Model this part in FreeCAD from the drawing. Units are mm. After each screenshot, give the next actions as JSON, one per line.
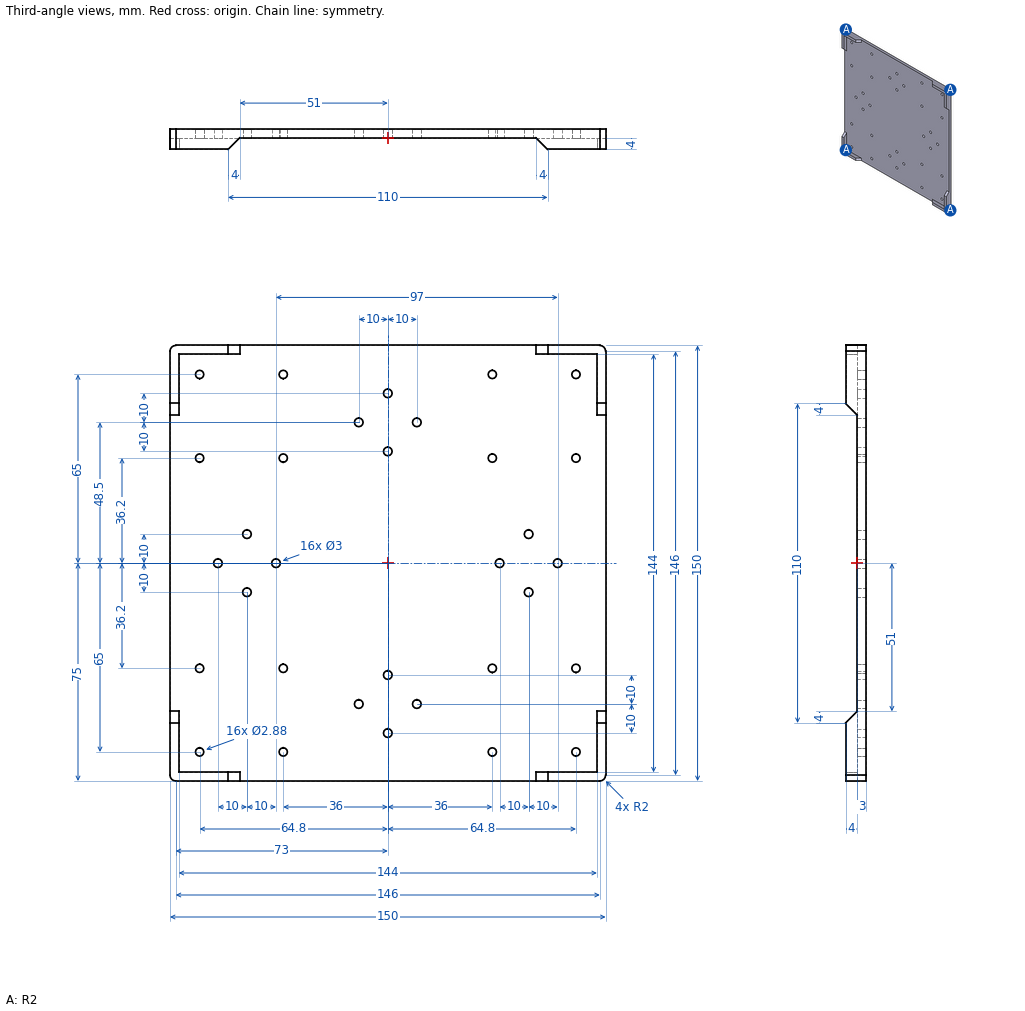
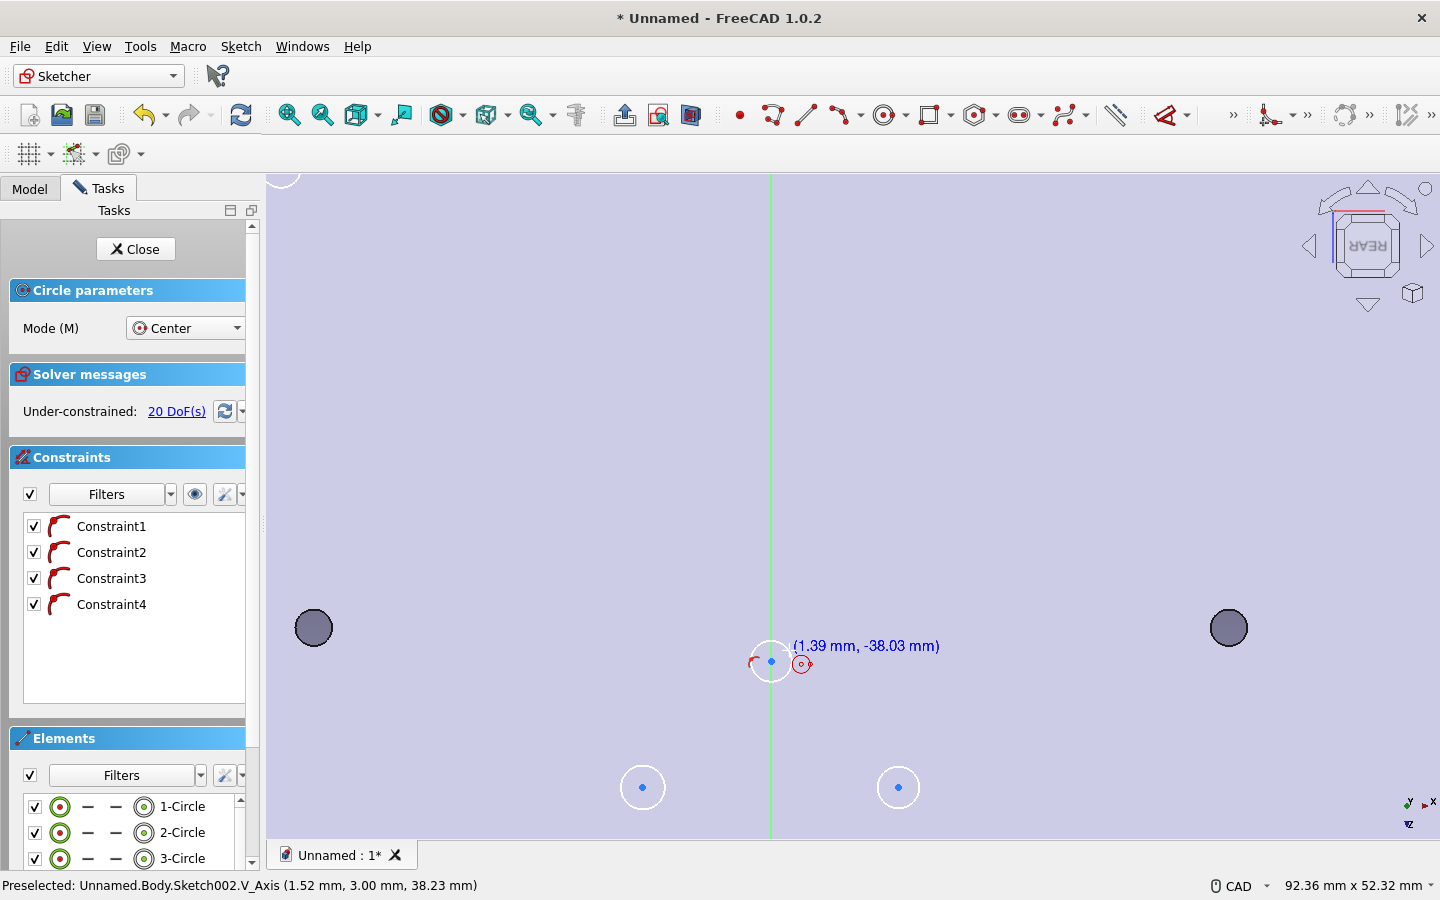
{"action": "scroll", "coordinate": [790, 653], "scroll_direction": "down", "scroll_amount": 6}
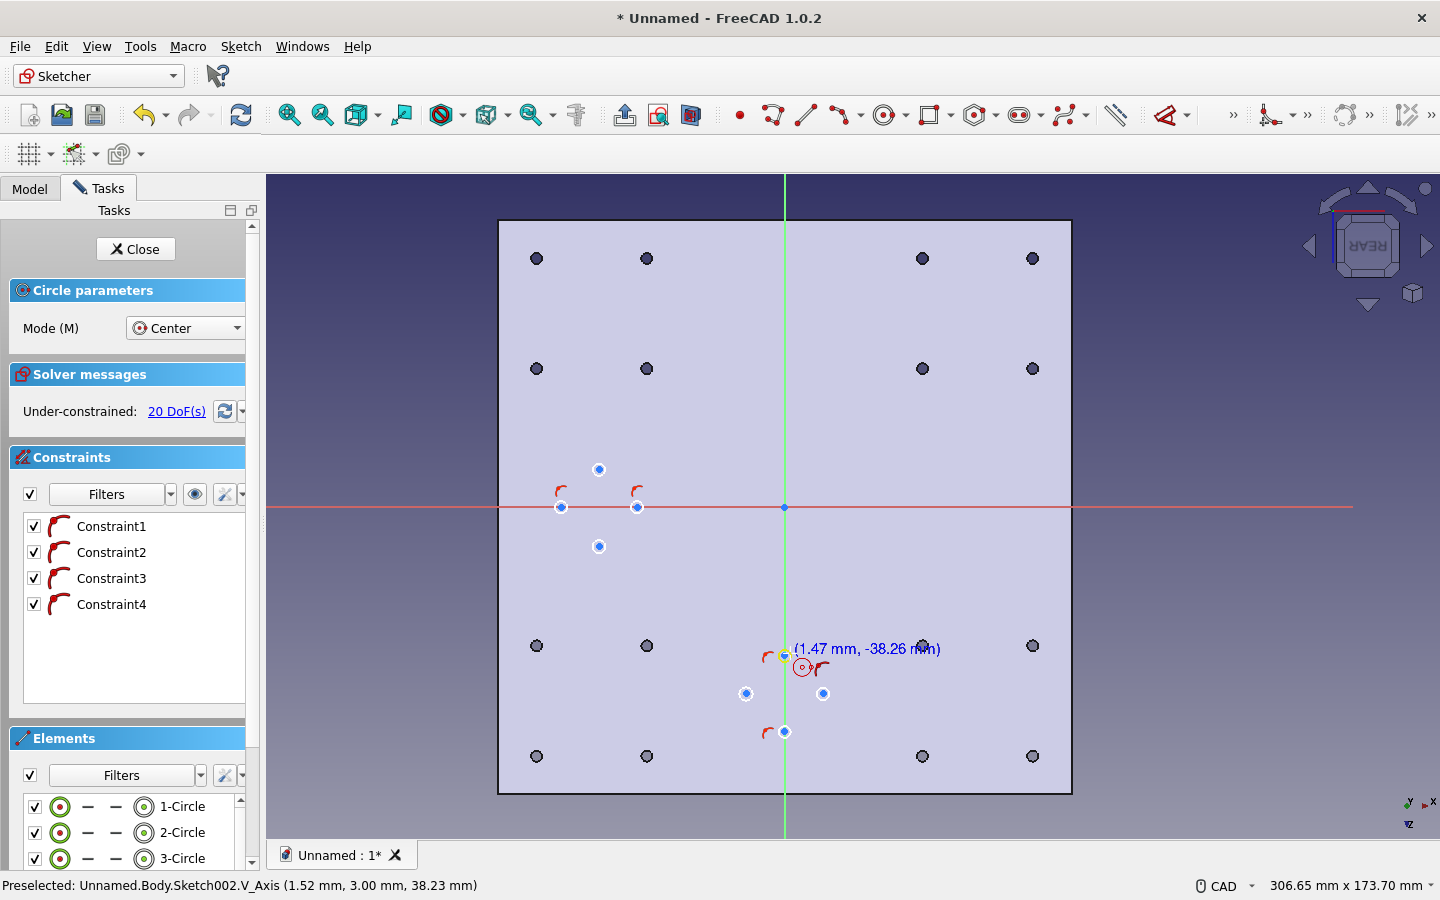
{"action": "scroll", "coordinate": [1009, 507], "scroll_direction": "up", "scroll_amount": 7}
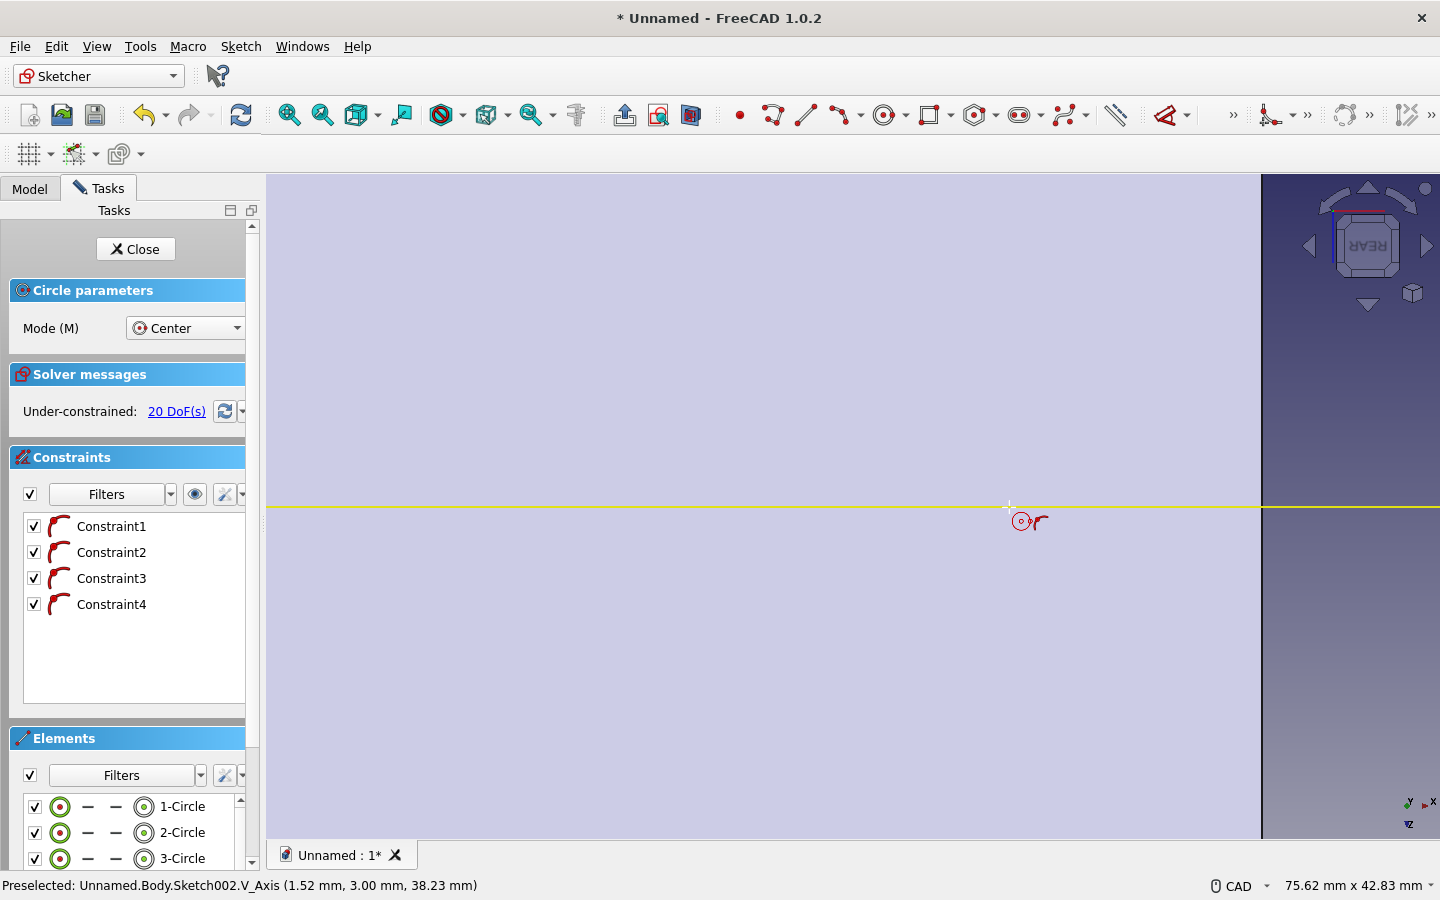
{"action": "scroll", "coordinate": [1009, 506], "scroll_direction": "down", "scroll_amount": 7}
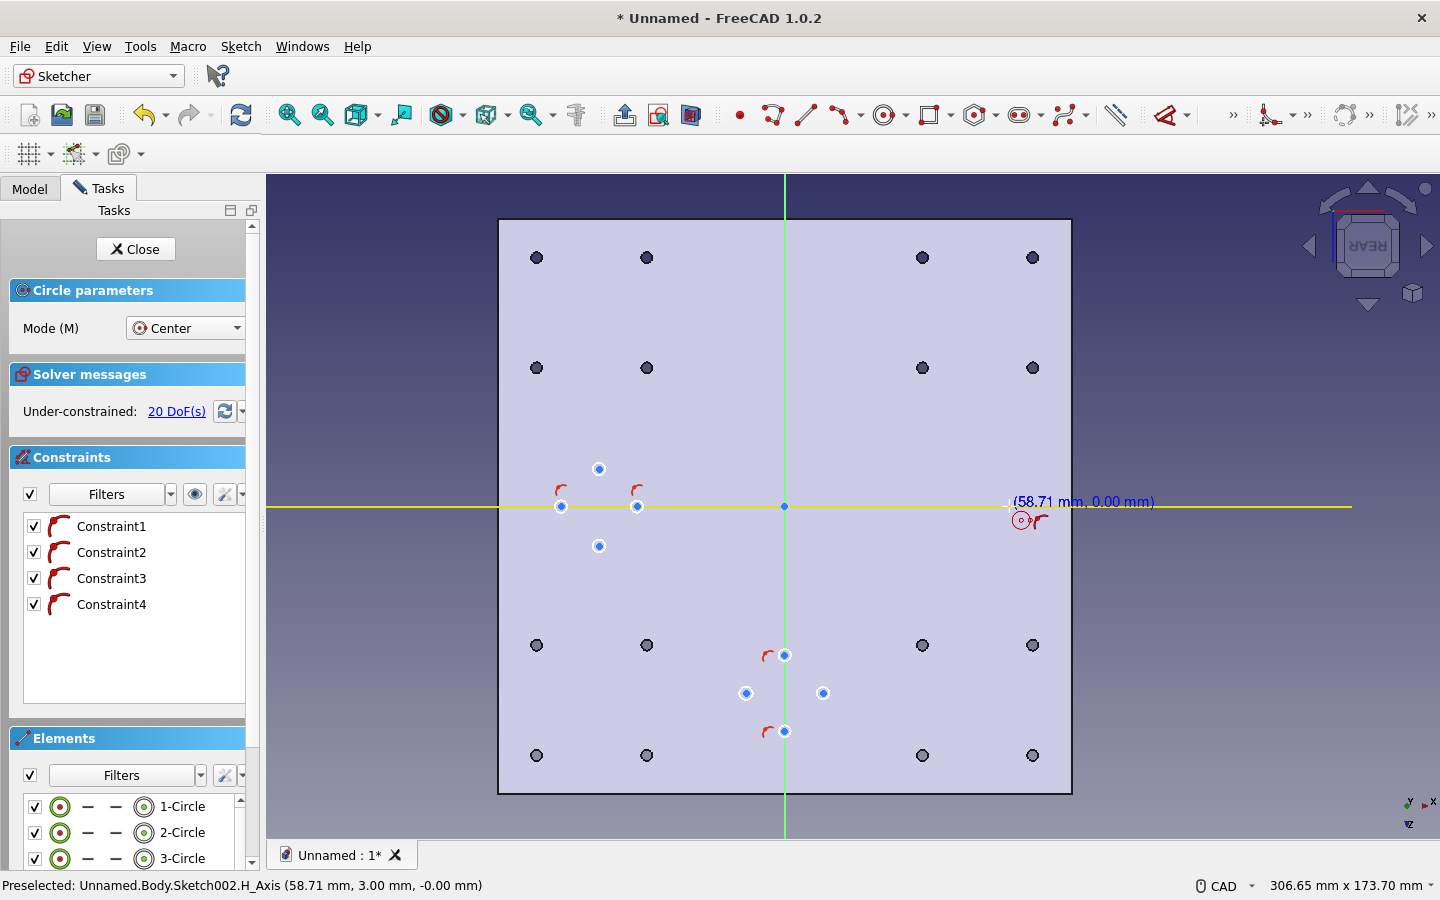
{"action": "left_click", "coordinate": [1009, 507]}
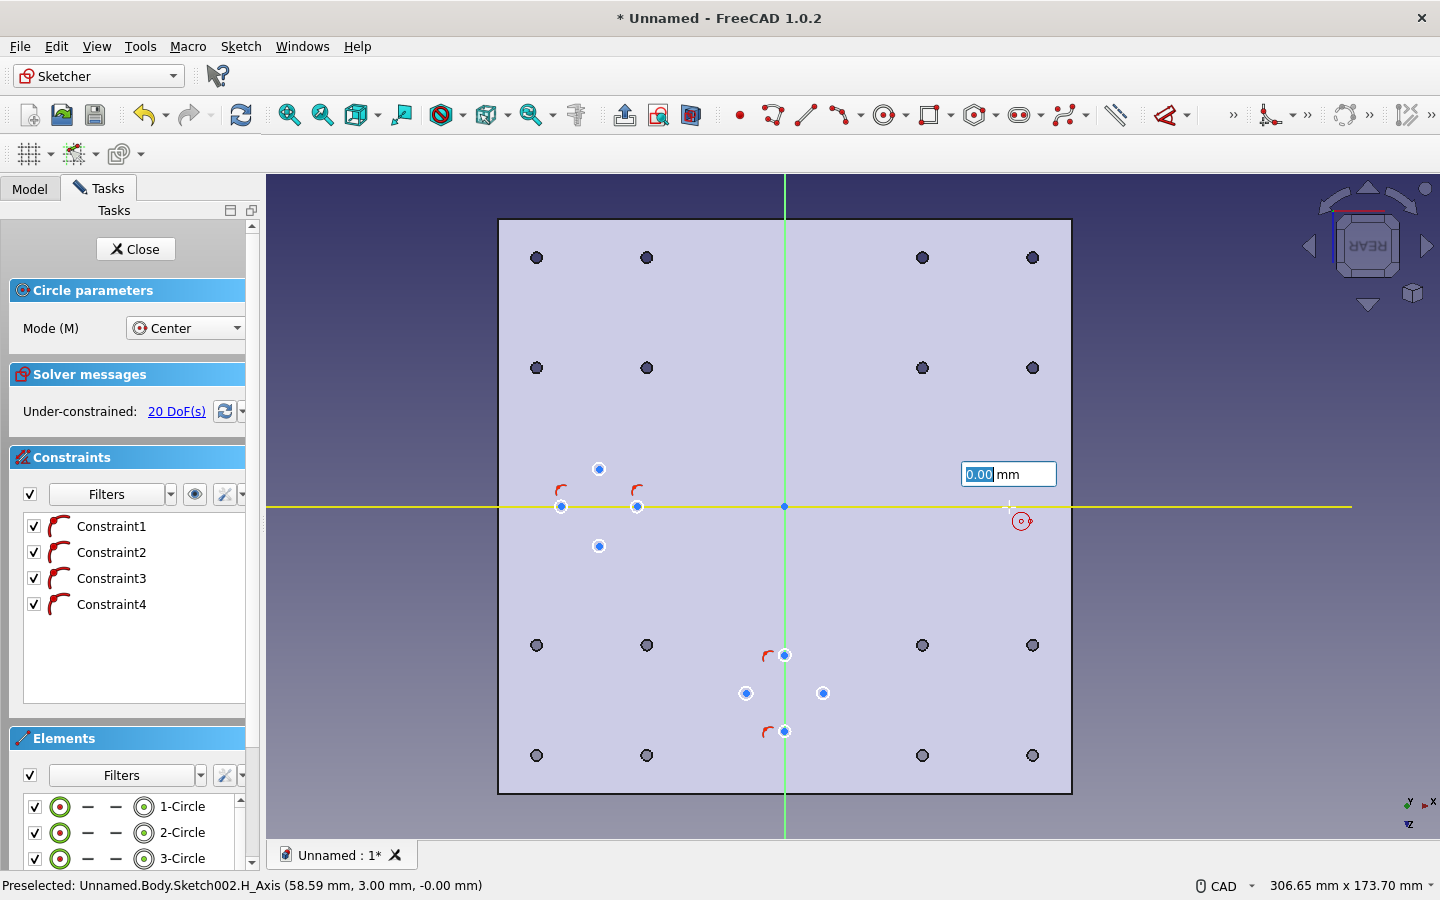
{"action": "scroll", "coordinate": [1007, 512], "scroll_direction": "up", "scroll_amount": 6}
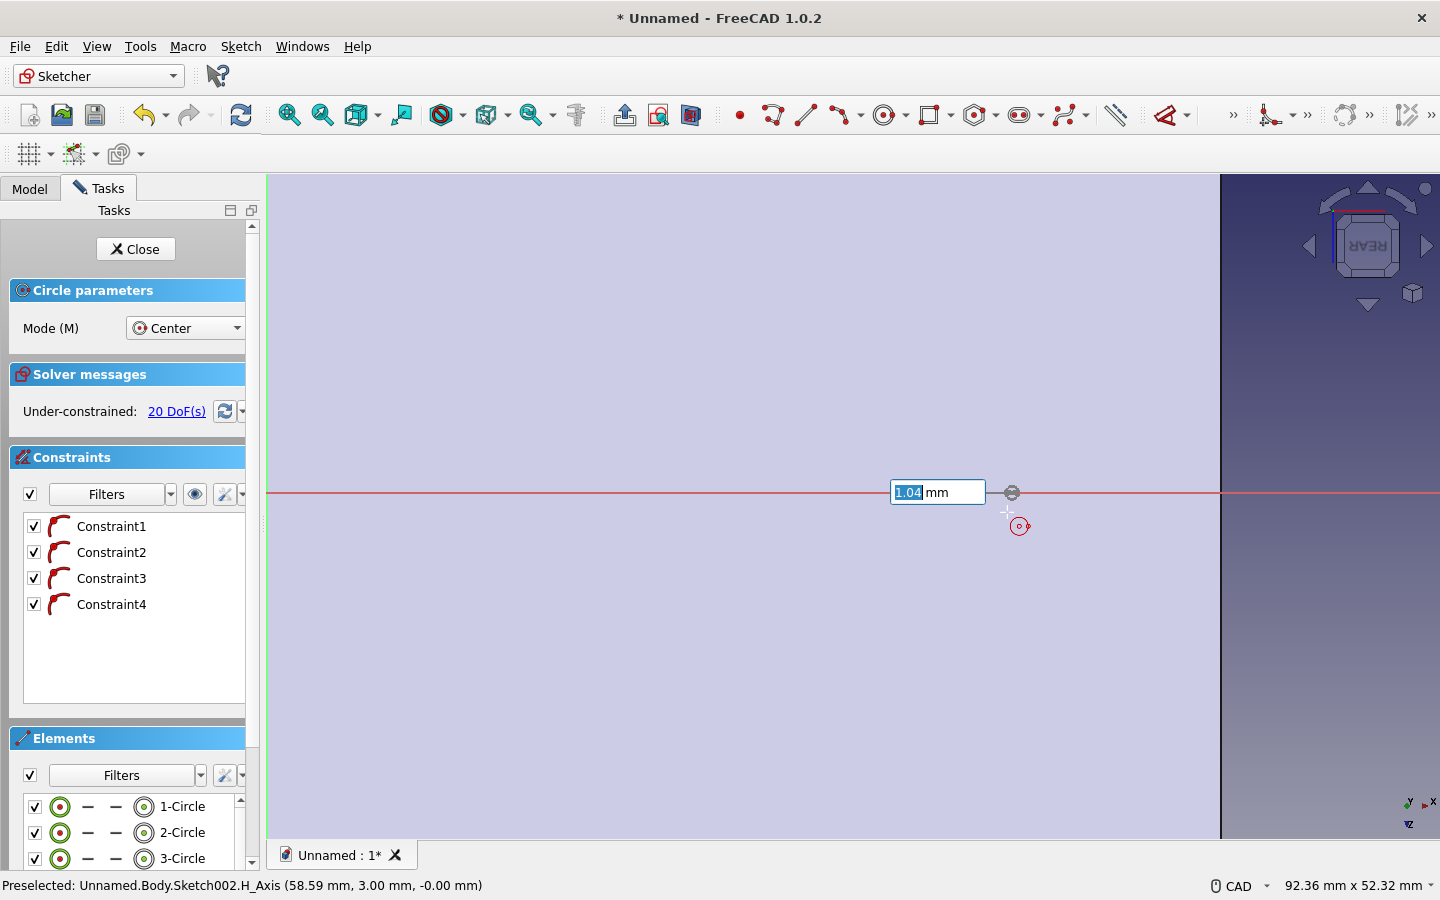
{"action": "left_click", "coordinate": [1005, 511]}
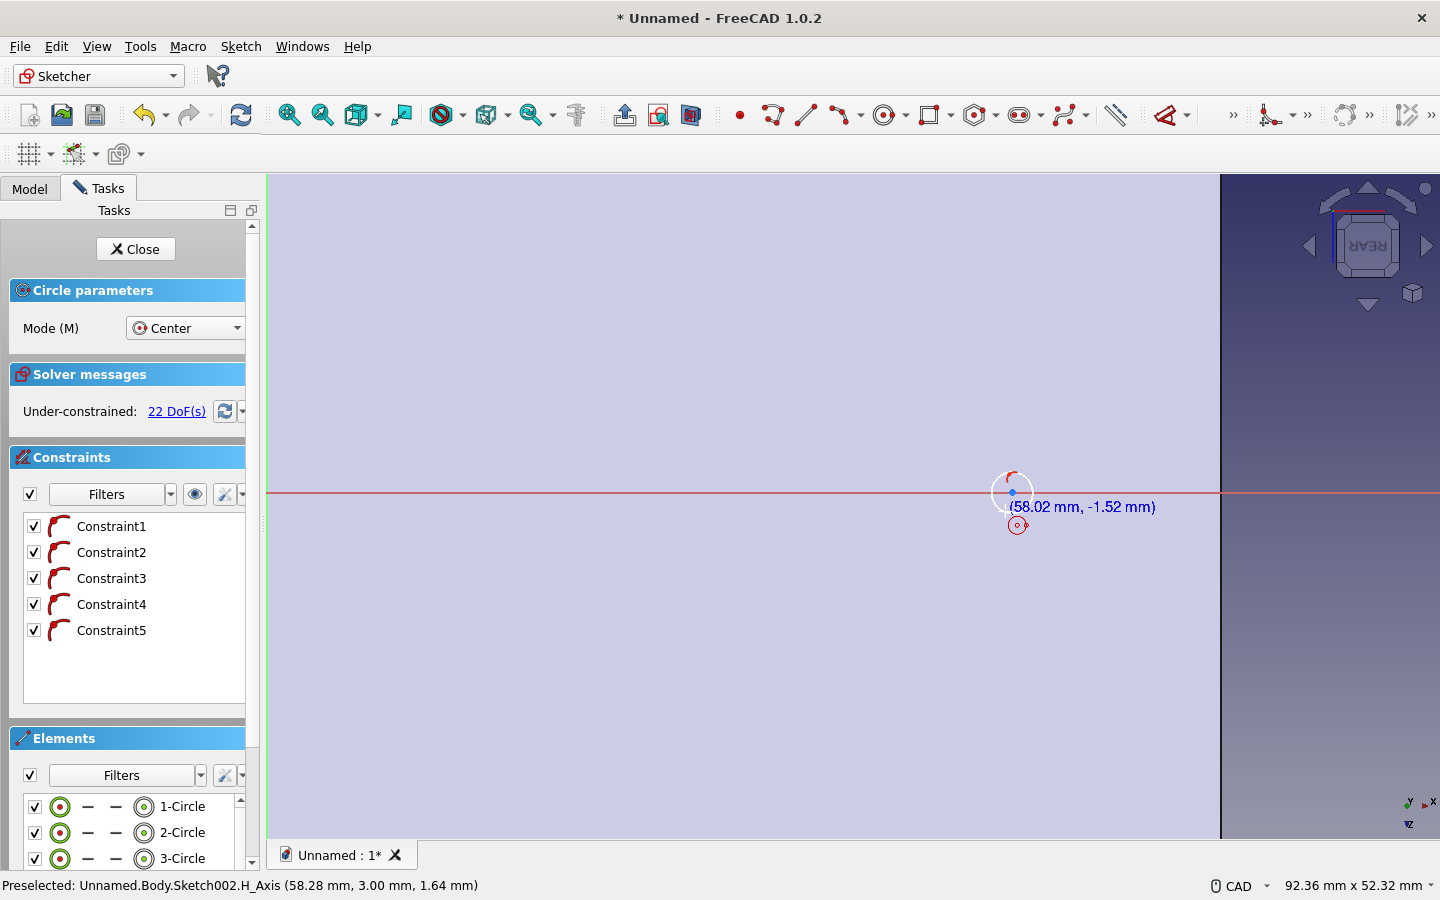
{"action": "scroll", "coordinate": [1007, 512], "scroll_direction": "down", "scroll_amount": 6}